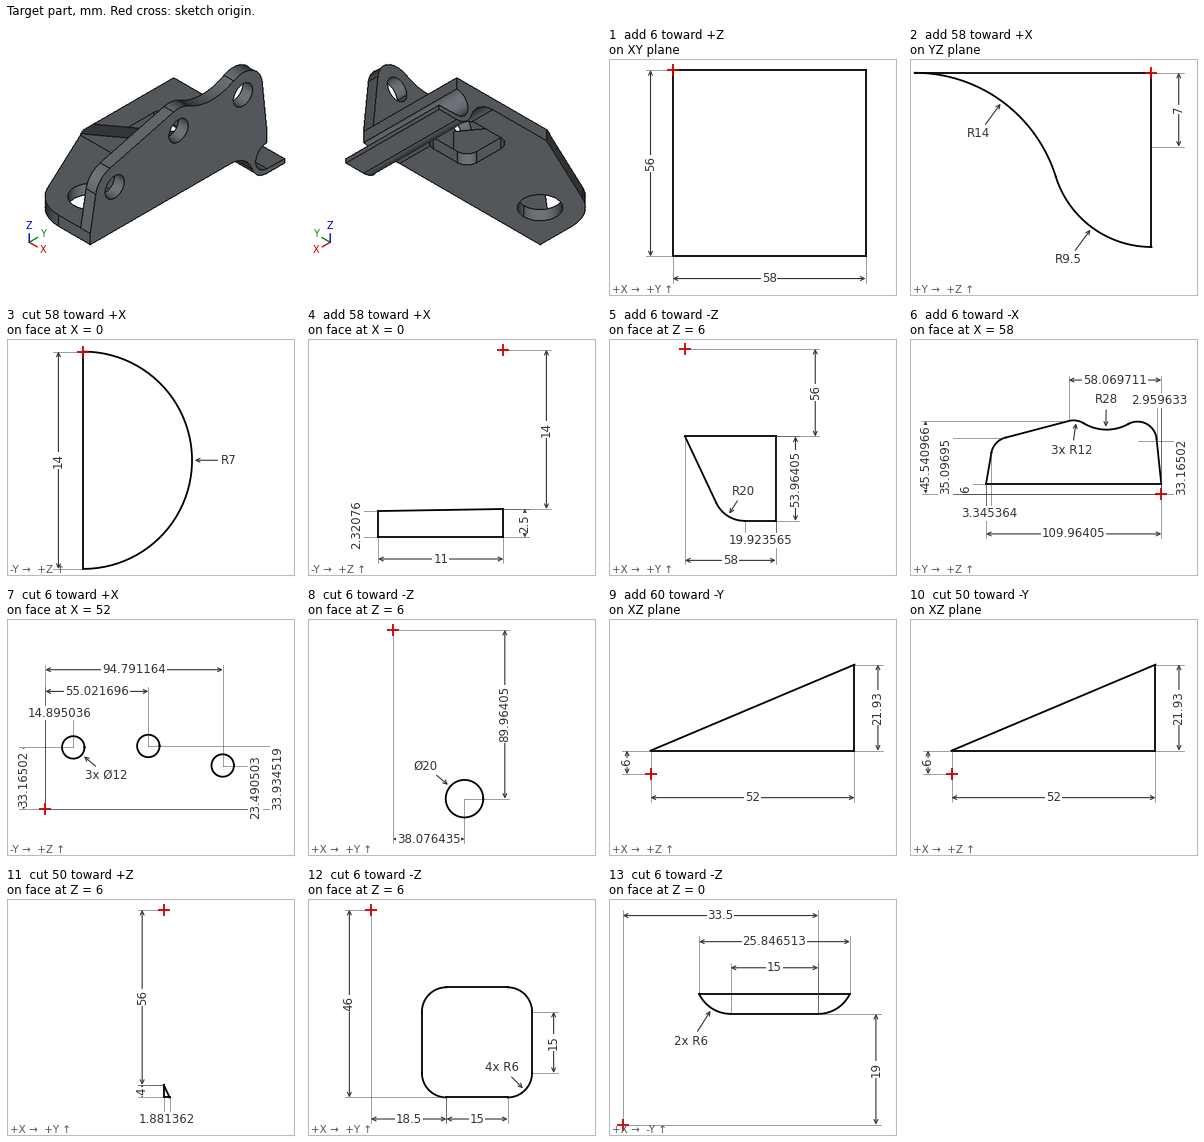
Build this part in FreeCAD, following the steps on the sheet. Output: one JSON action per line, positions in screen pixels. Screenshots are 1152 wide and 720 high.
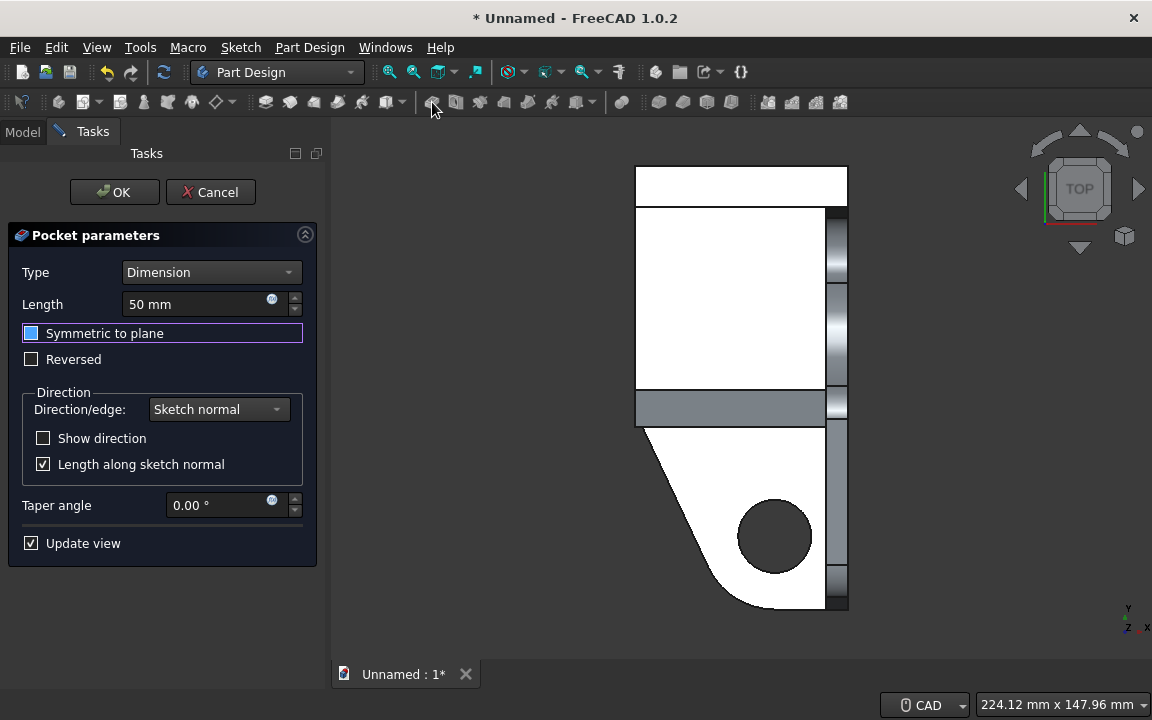
{"action": "left_click", "coordinate": [30, 359]}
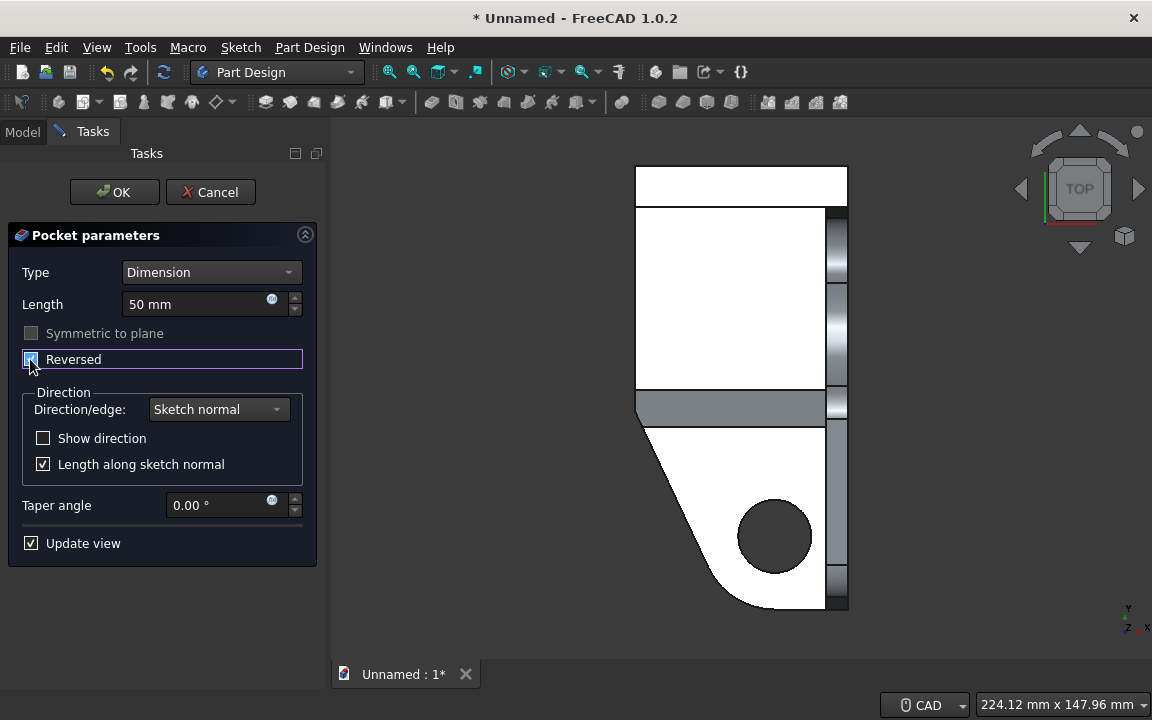
{"action": "left_click", "coordinate": [115, 192]}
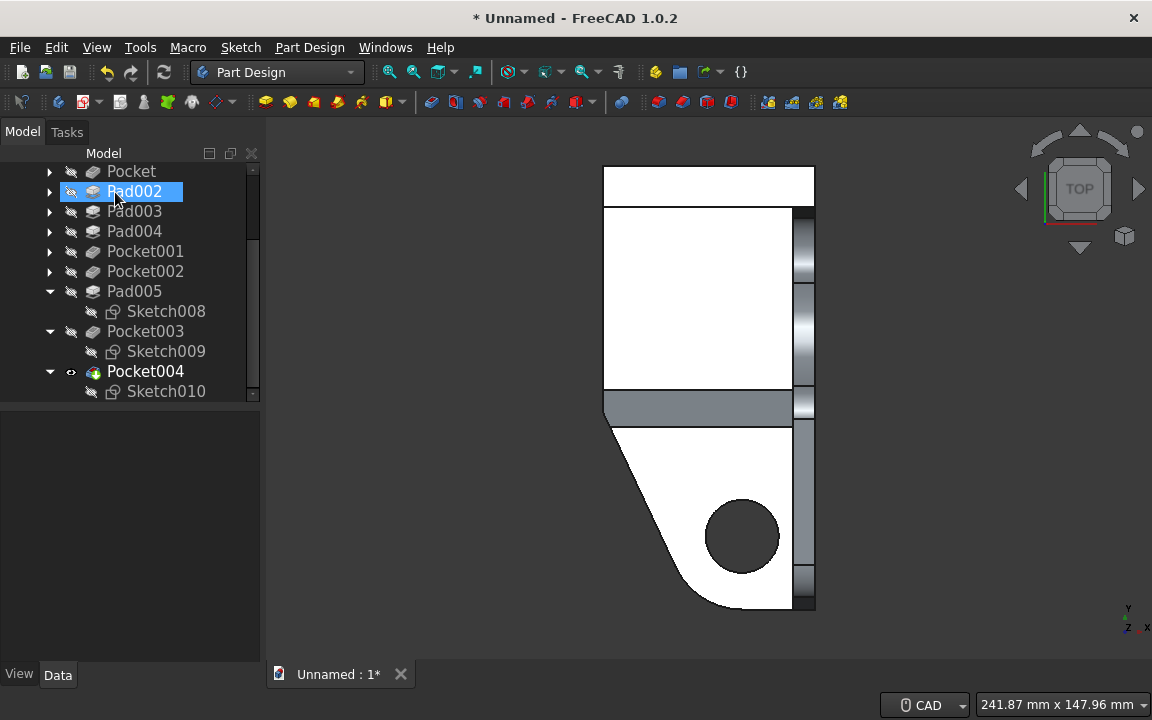
{"action": "left_click", "coordinate": [698, 297]}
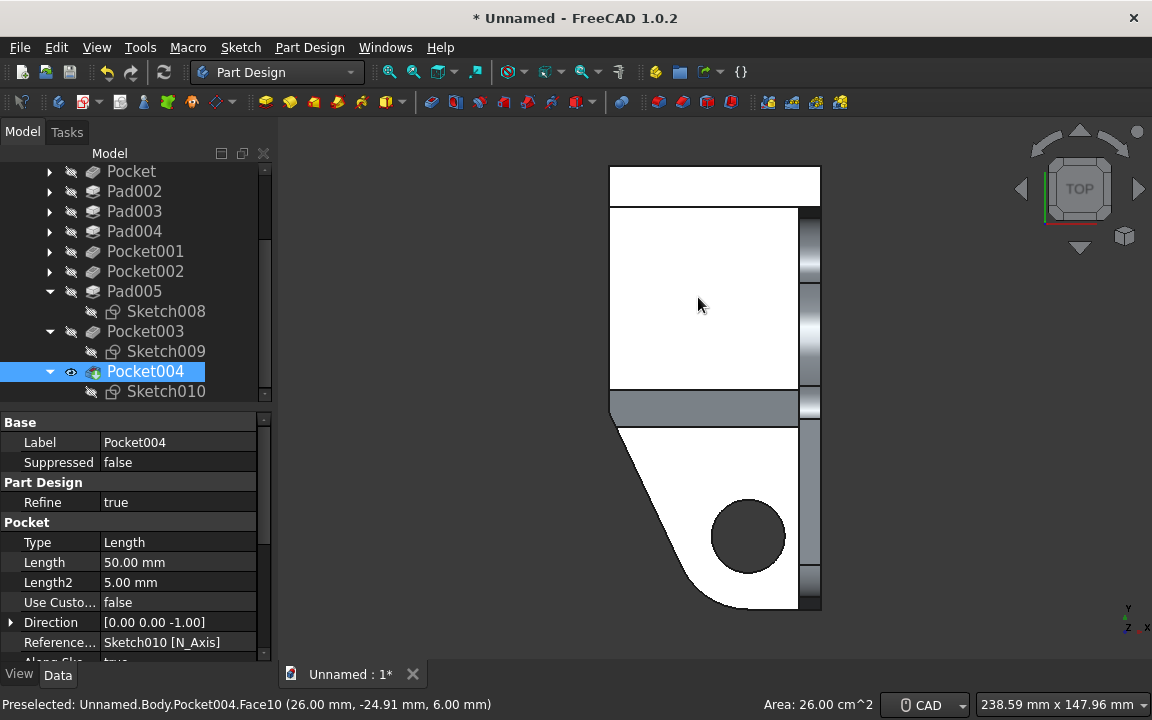
{"action": "left_click", "coordinate": [84, 102]}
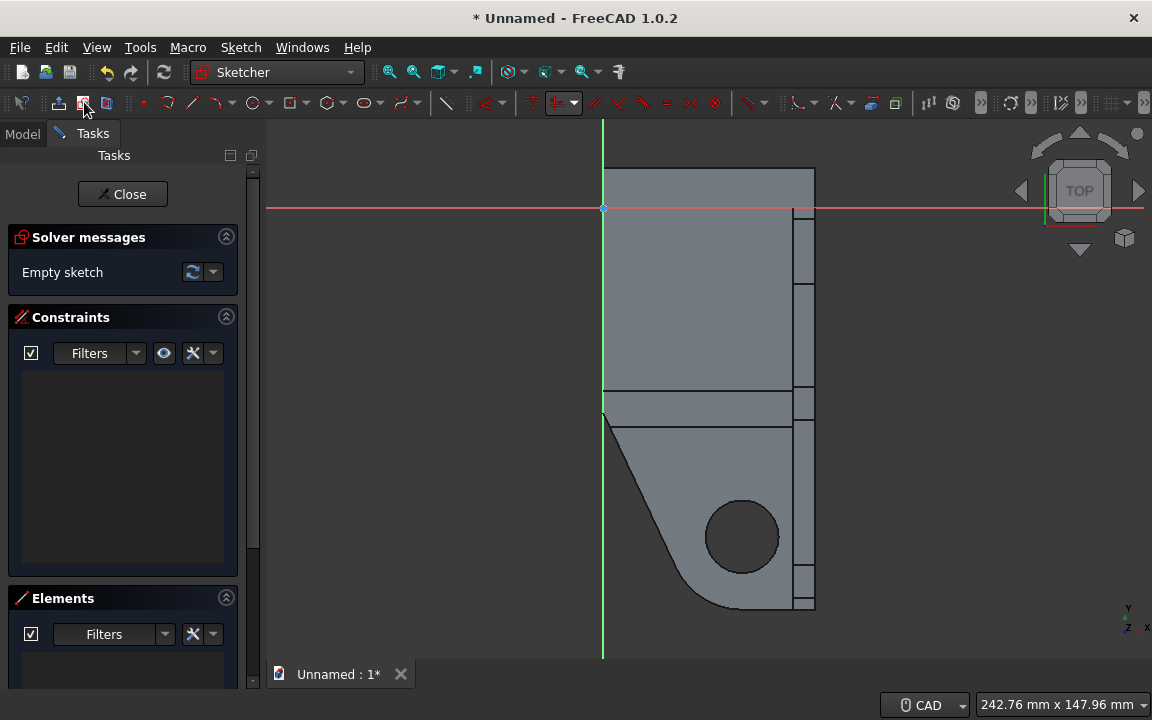
{"action": "scroll", "coordinate": [704, 213], "scroll_direction": "up", "scroll_amount": 4}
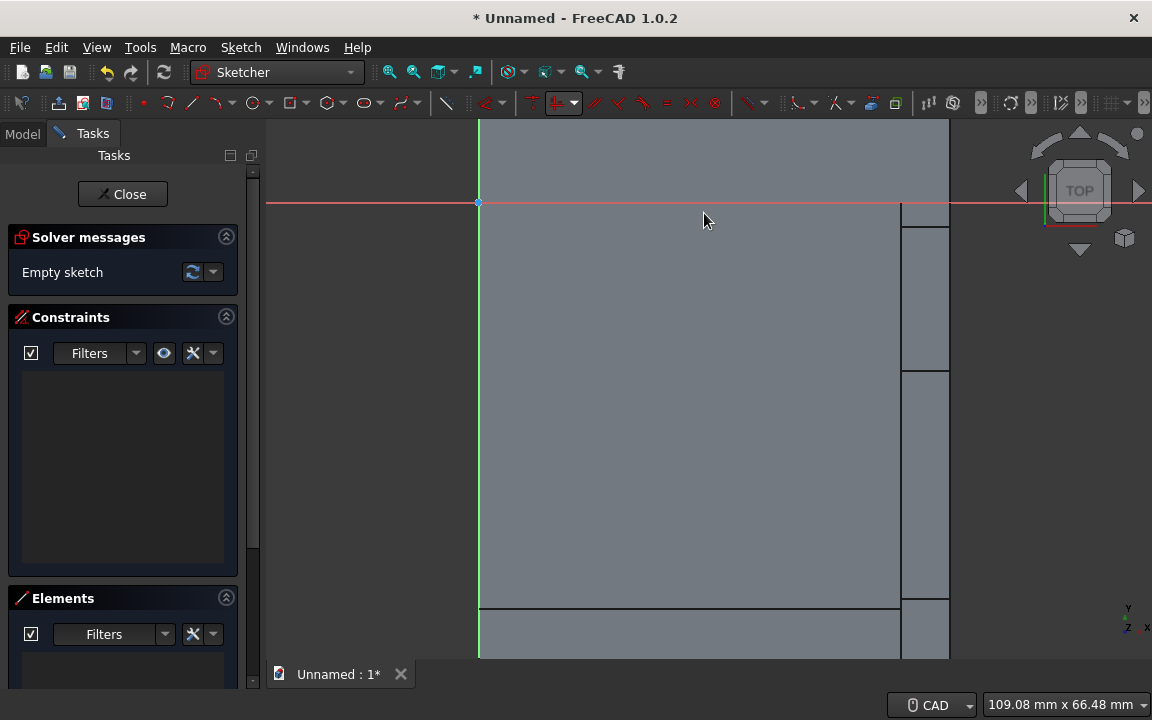
{"action": "left_click", "coordinate": [192, 104]}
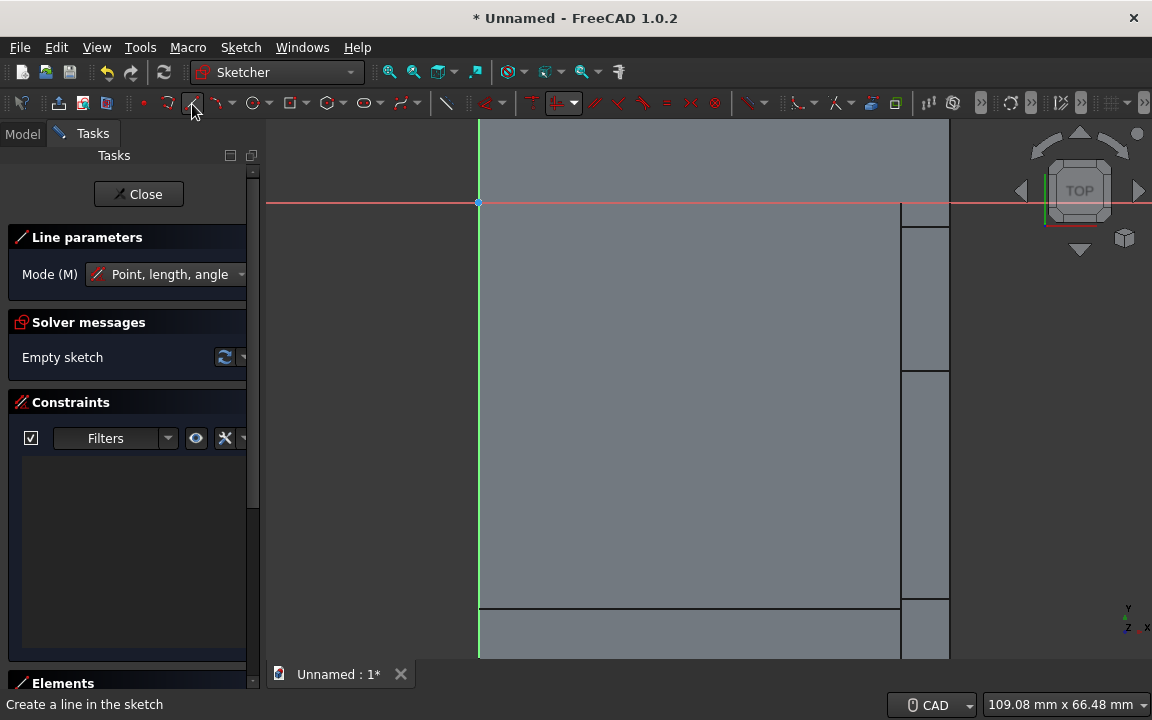
{"action": "left_click", "coordinate": [629, 576]}
{"action": "left_click", "coordinate": [751, 576]}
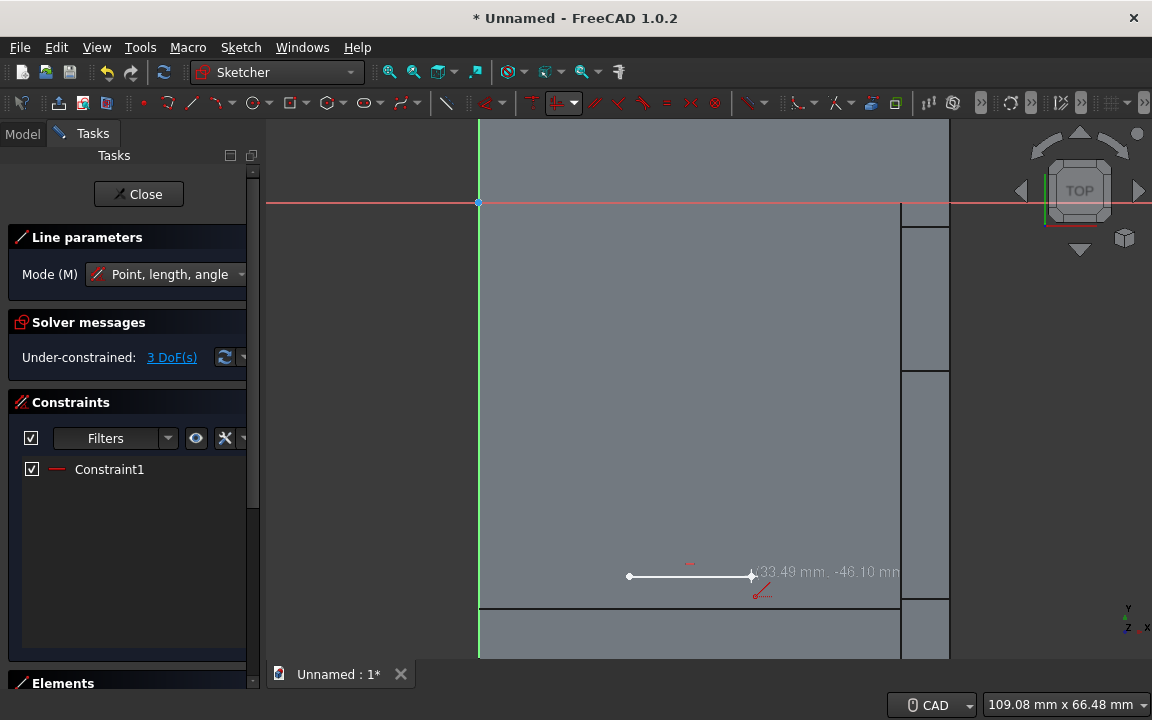
{"action": "left_click", "coordinate": [800, 527]}
{"action": "left_click", "coordinate": [800, 406]}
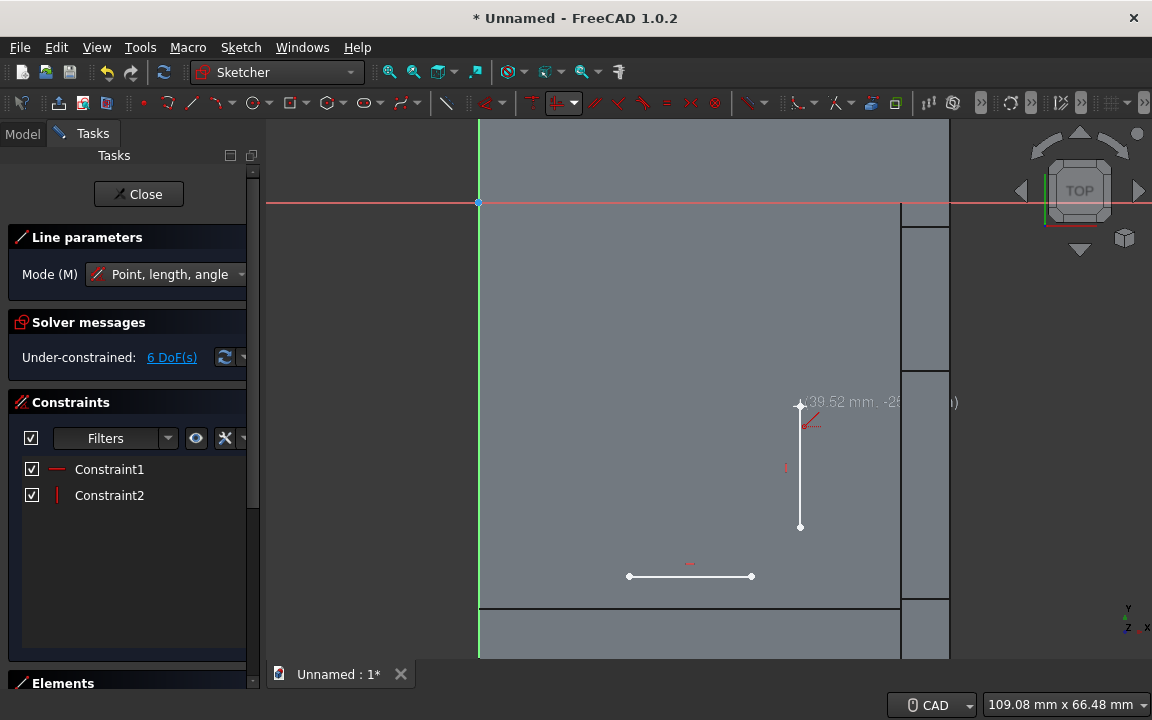
{"action": "left_click", "coordinate": [751, 357]}
{"action": "left_click", "coordinate": [629, 357]}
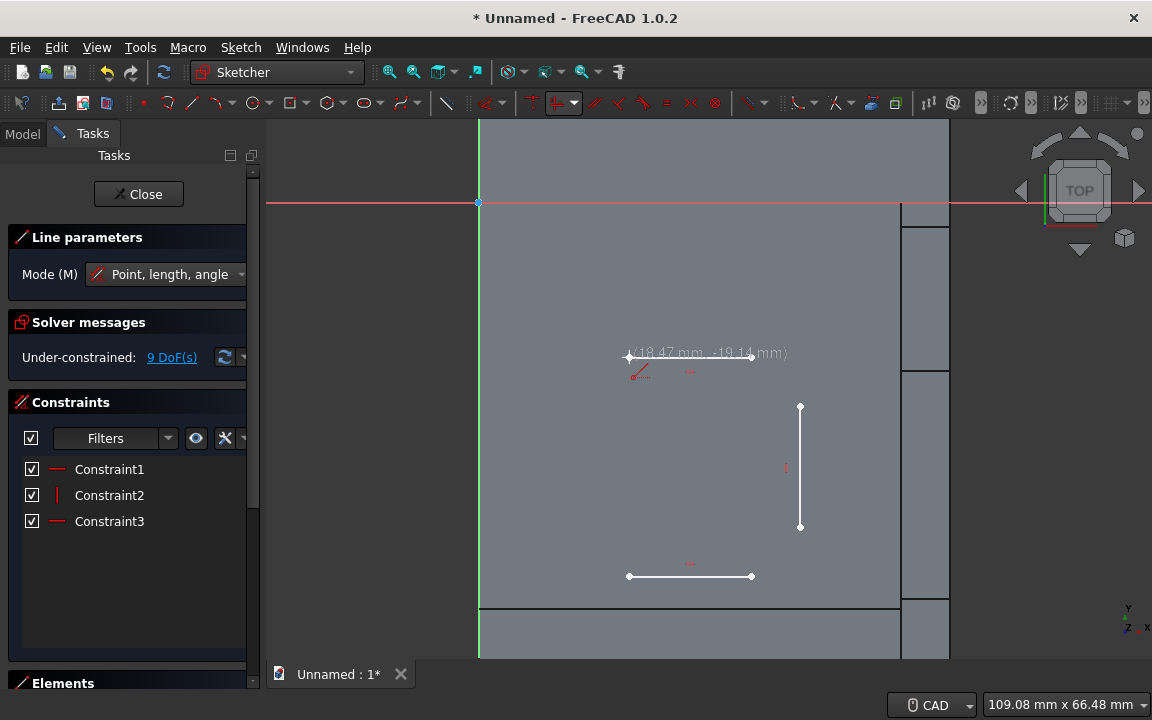
{"action": "left_click", "coordinate": [581, 406]}
{"action": "left_click", "coordinate": [581, 527]}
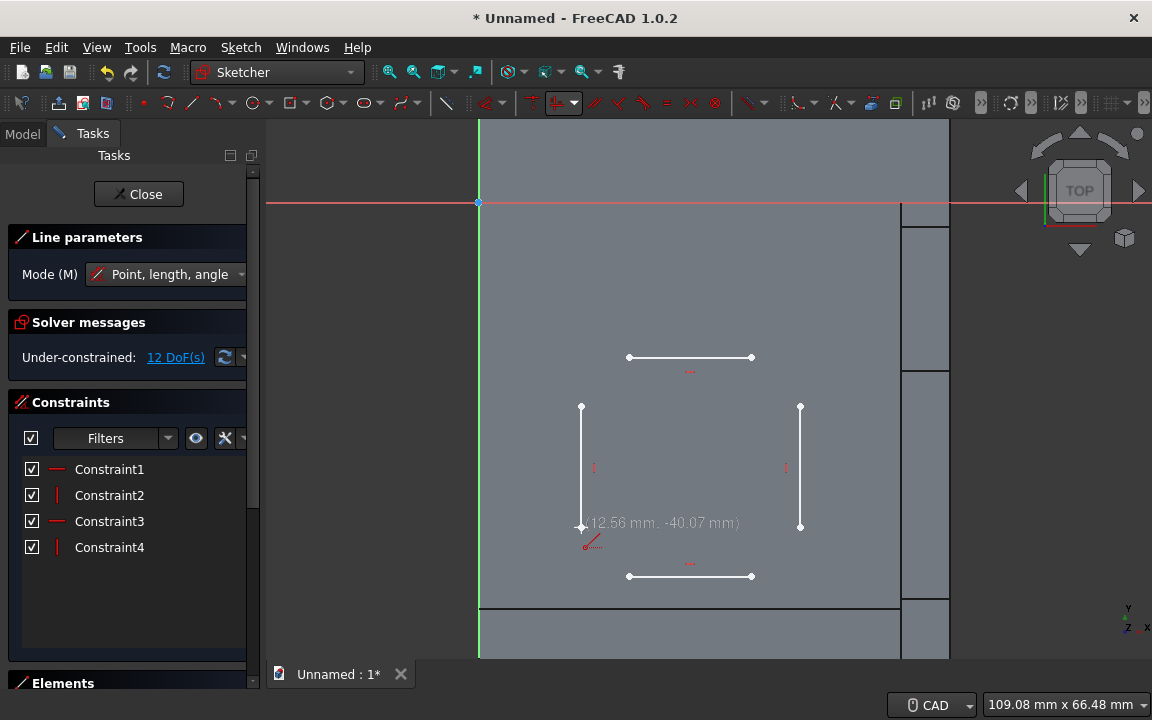
{"action": "left_click", "coordinate": [216, 104]}